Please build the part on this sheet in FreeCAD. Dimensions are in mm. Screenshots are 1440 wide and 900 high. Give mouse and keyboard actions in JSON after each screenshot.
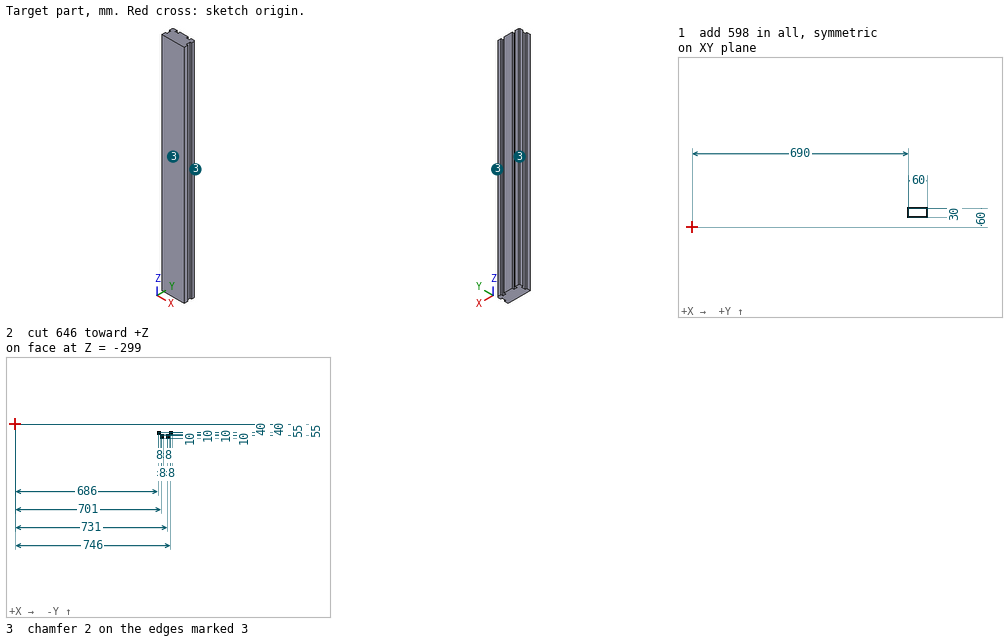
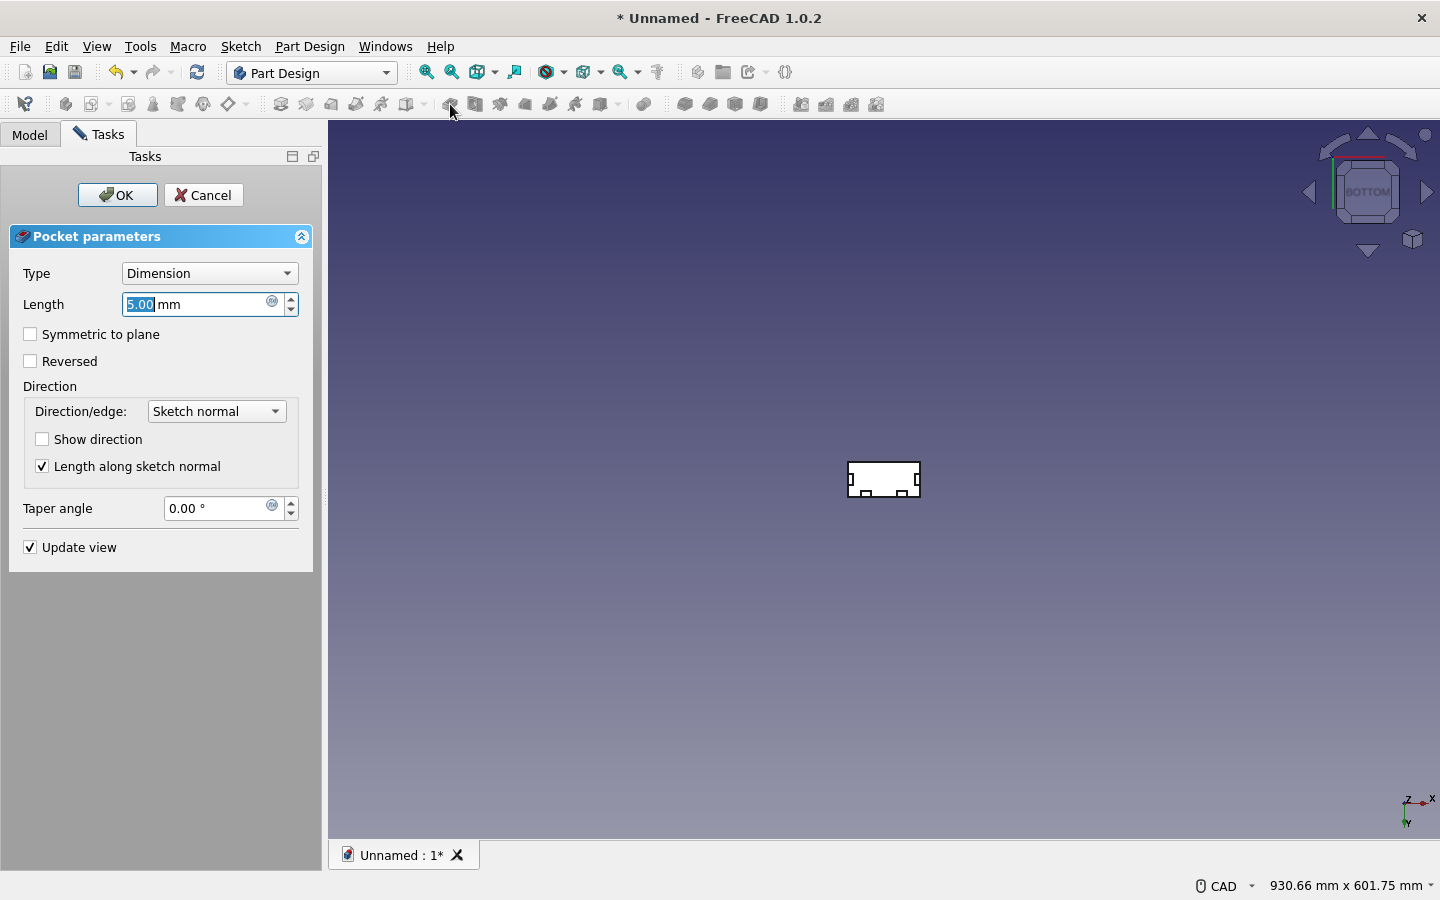
{"action": "type", "text": "646"}
{"action": "key", "text": "Tab"}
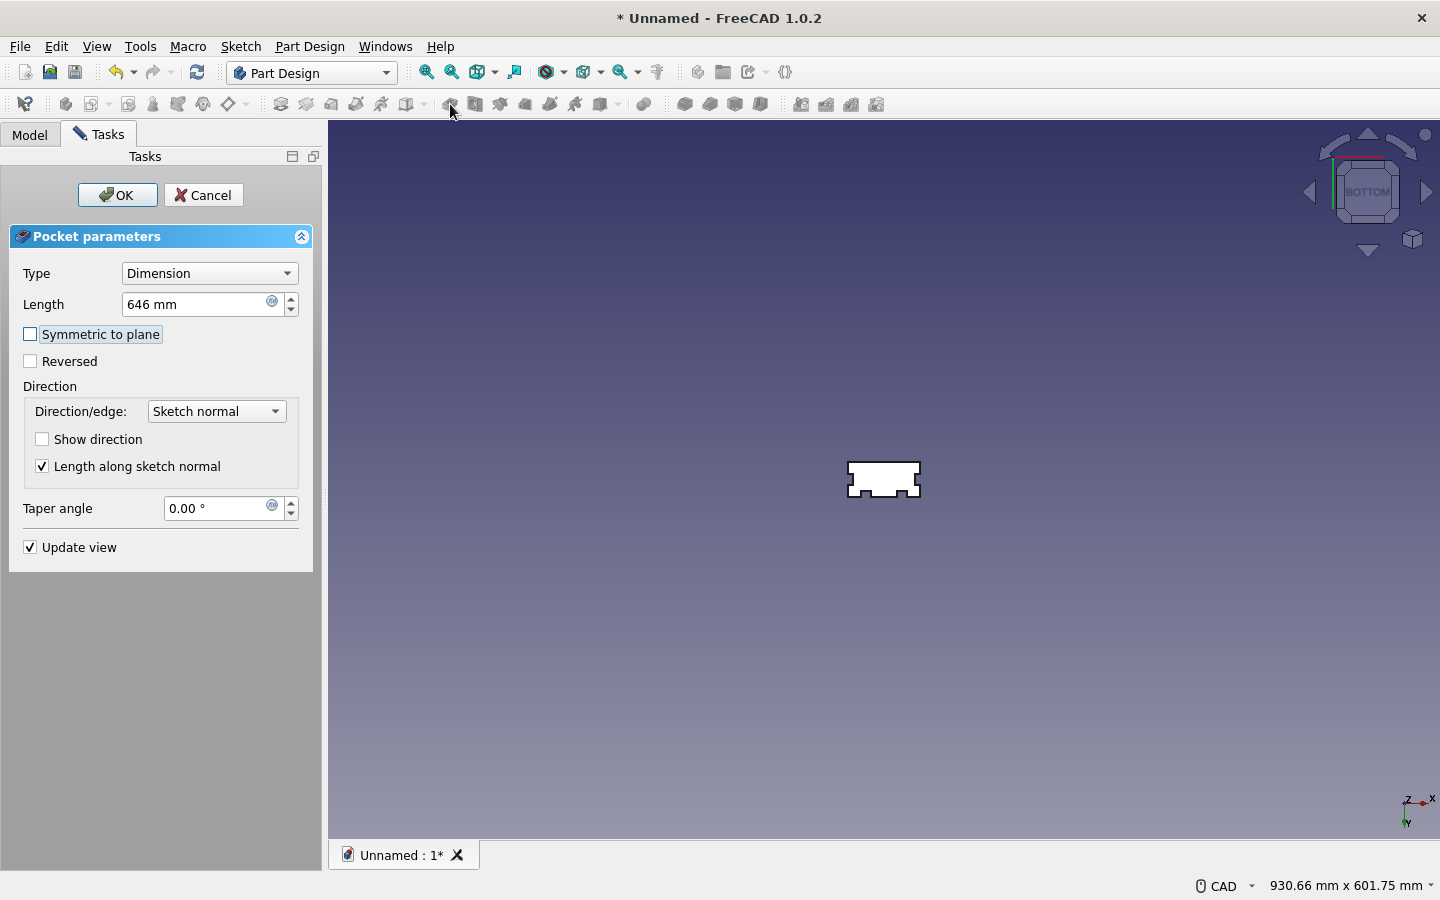
{"action": "left_click", "coordinate": [118, 195]}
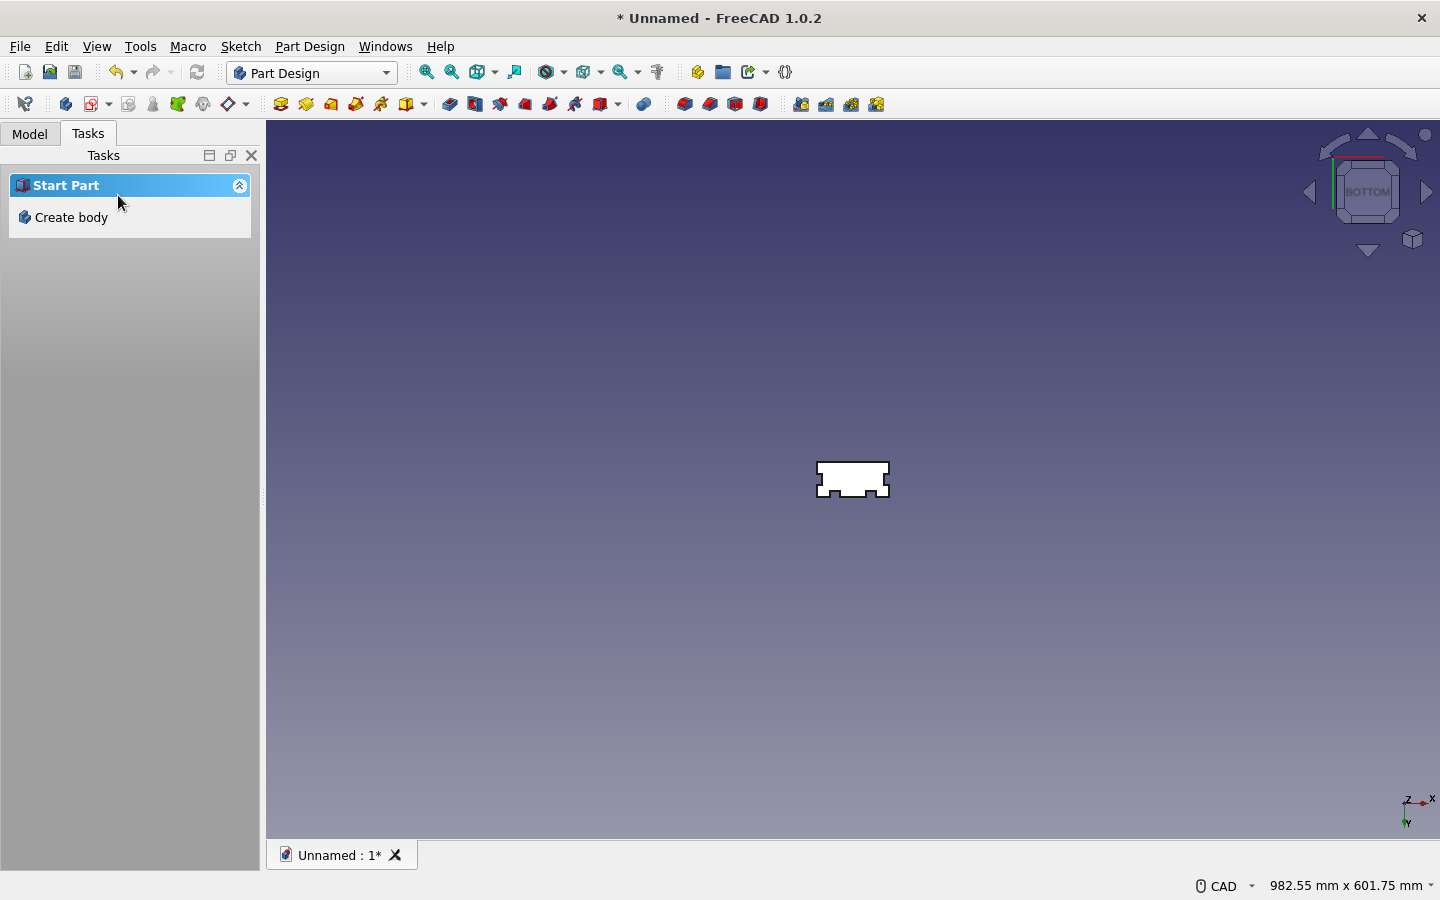
{"action": "left_click", "coordinate": [427, 72]}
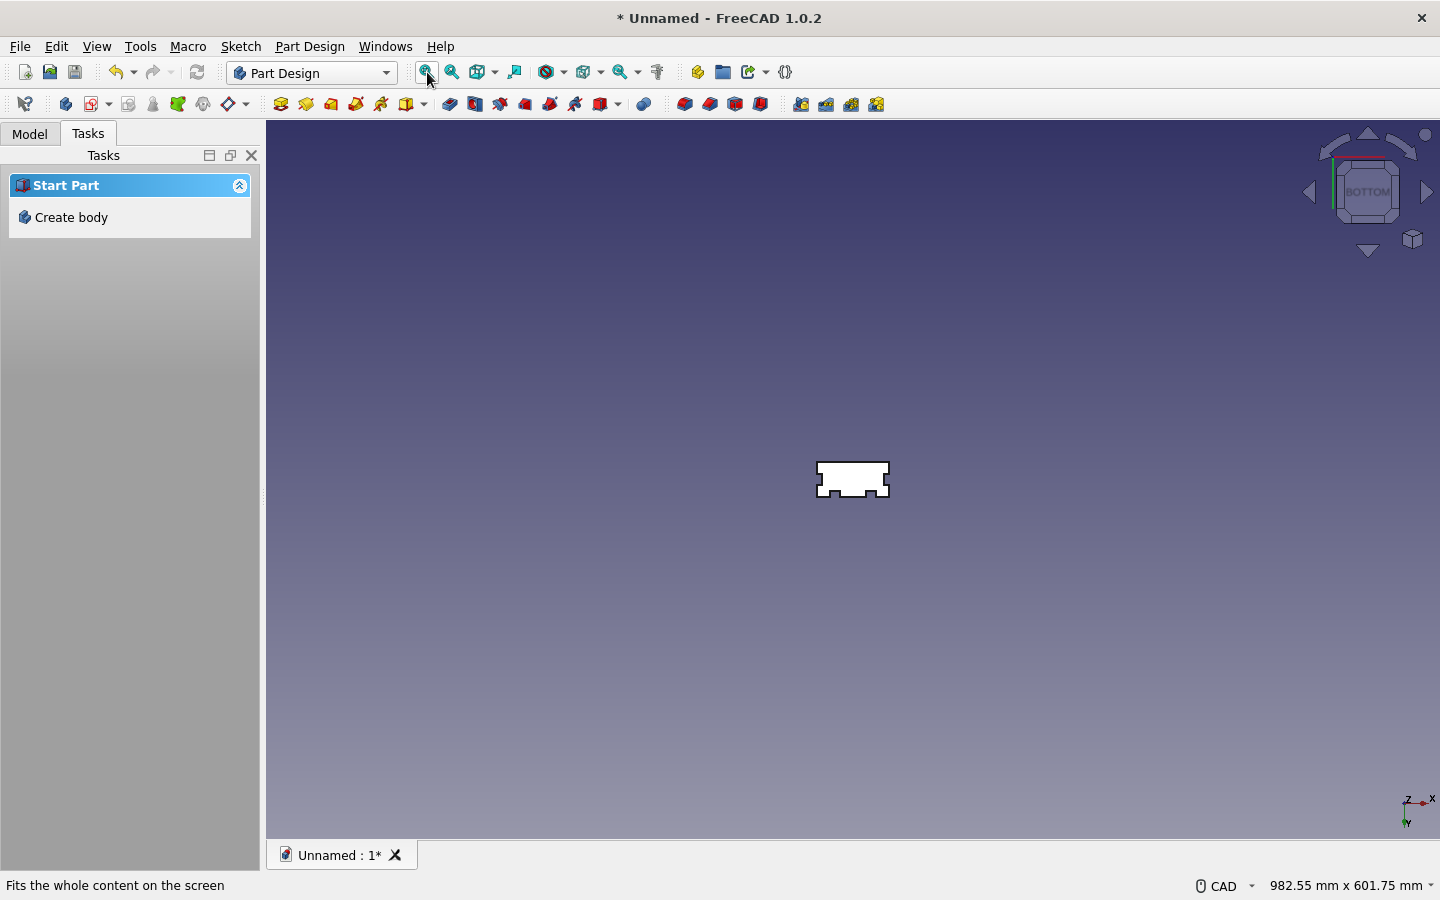
{"action": "key", "text": "0"}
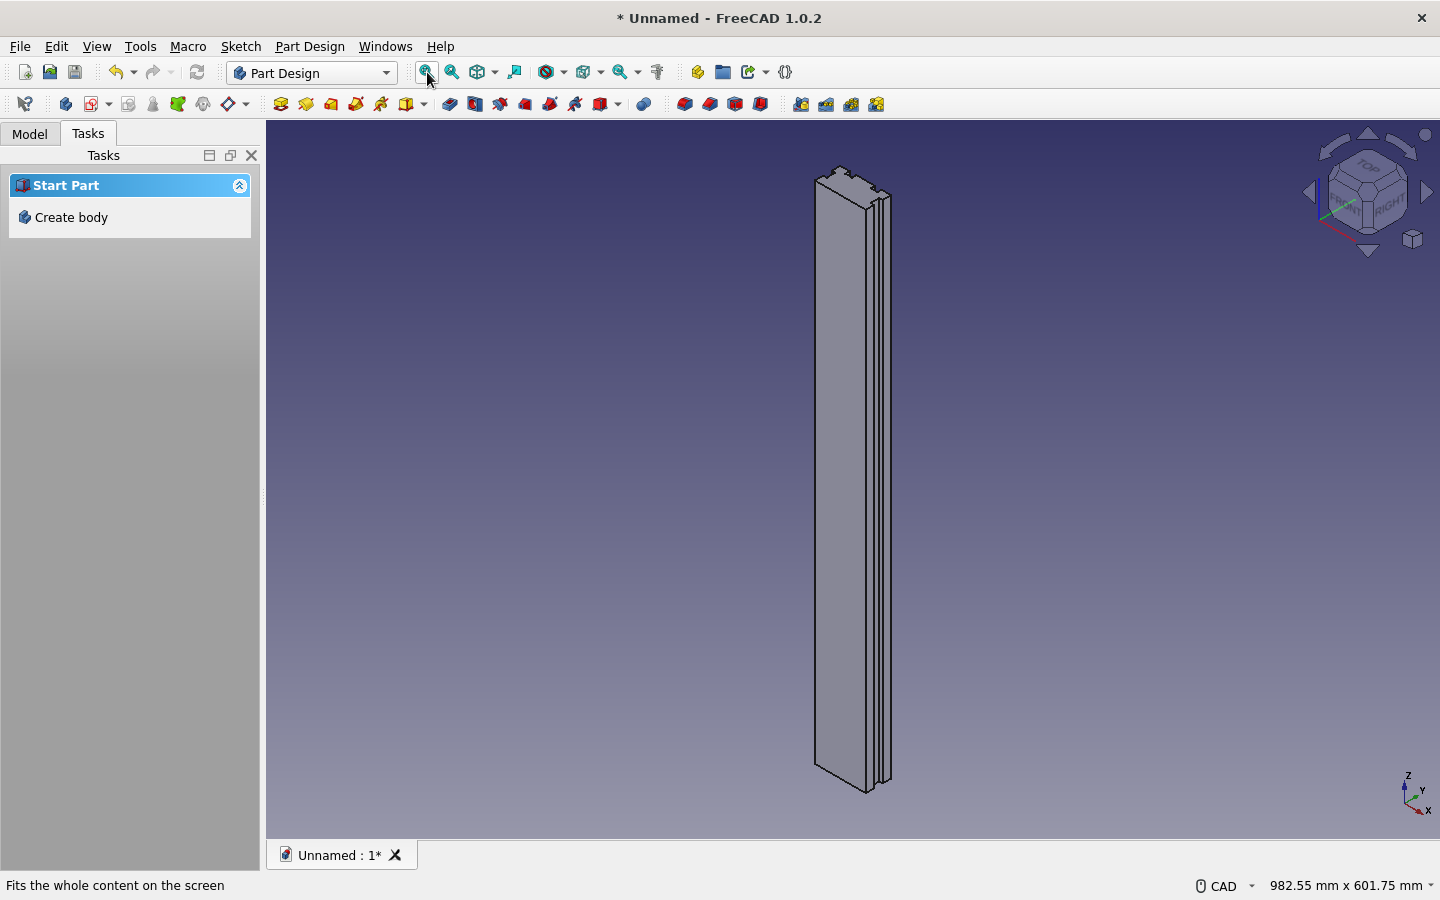
{"action": "key", "text": "2"}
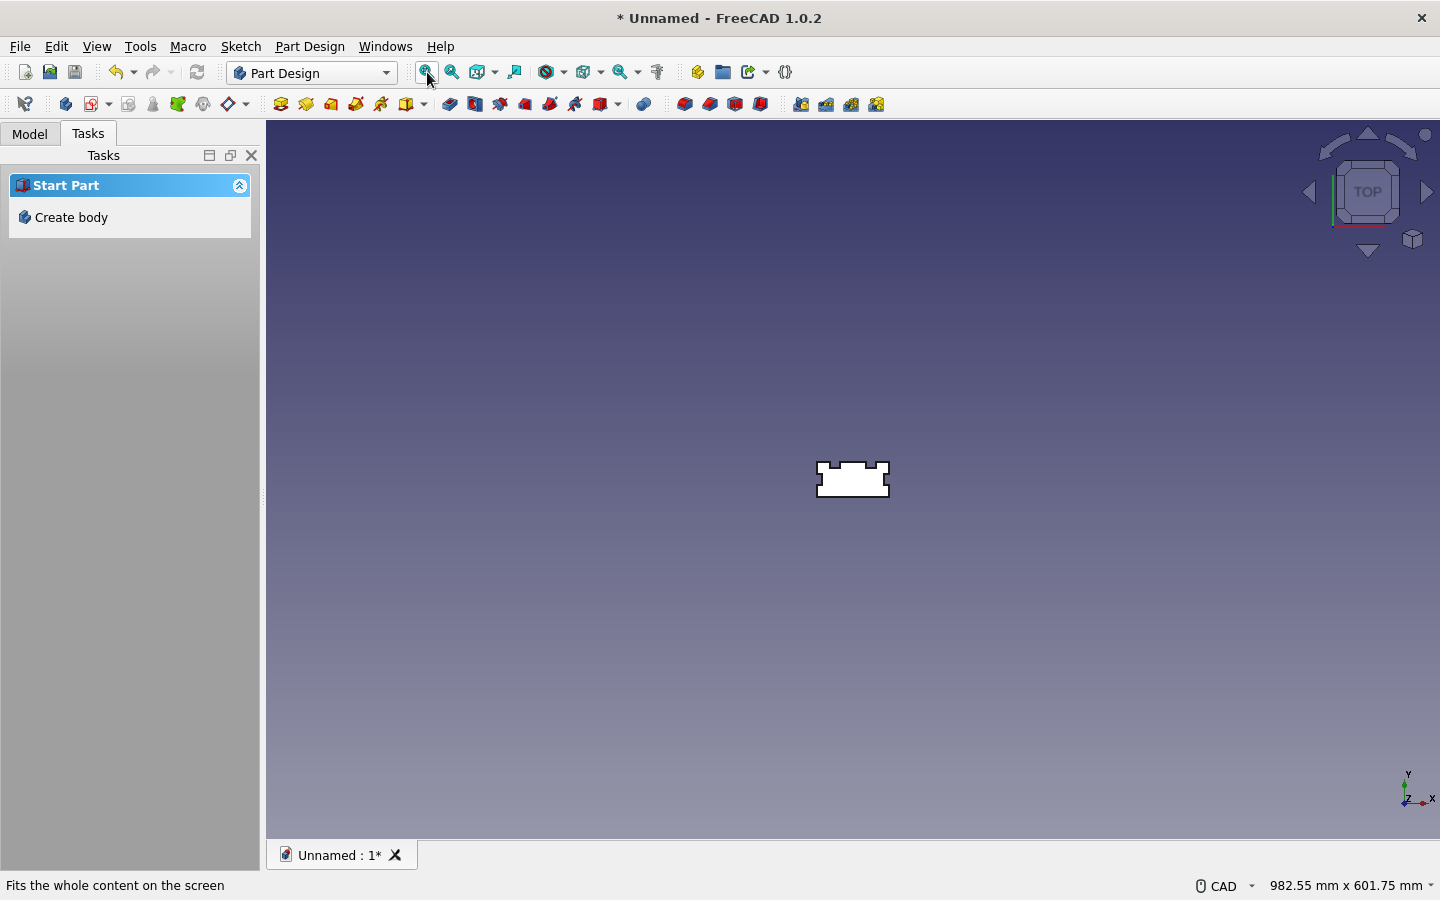
{"action": "key", "text": "v f"}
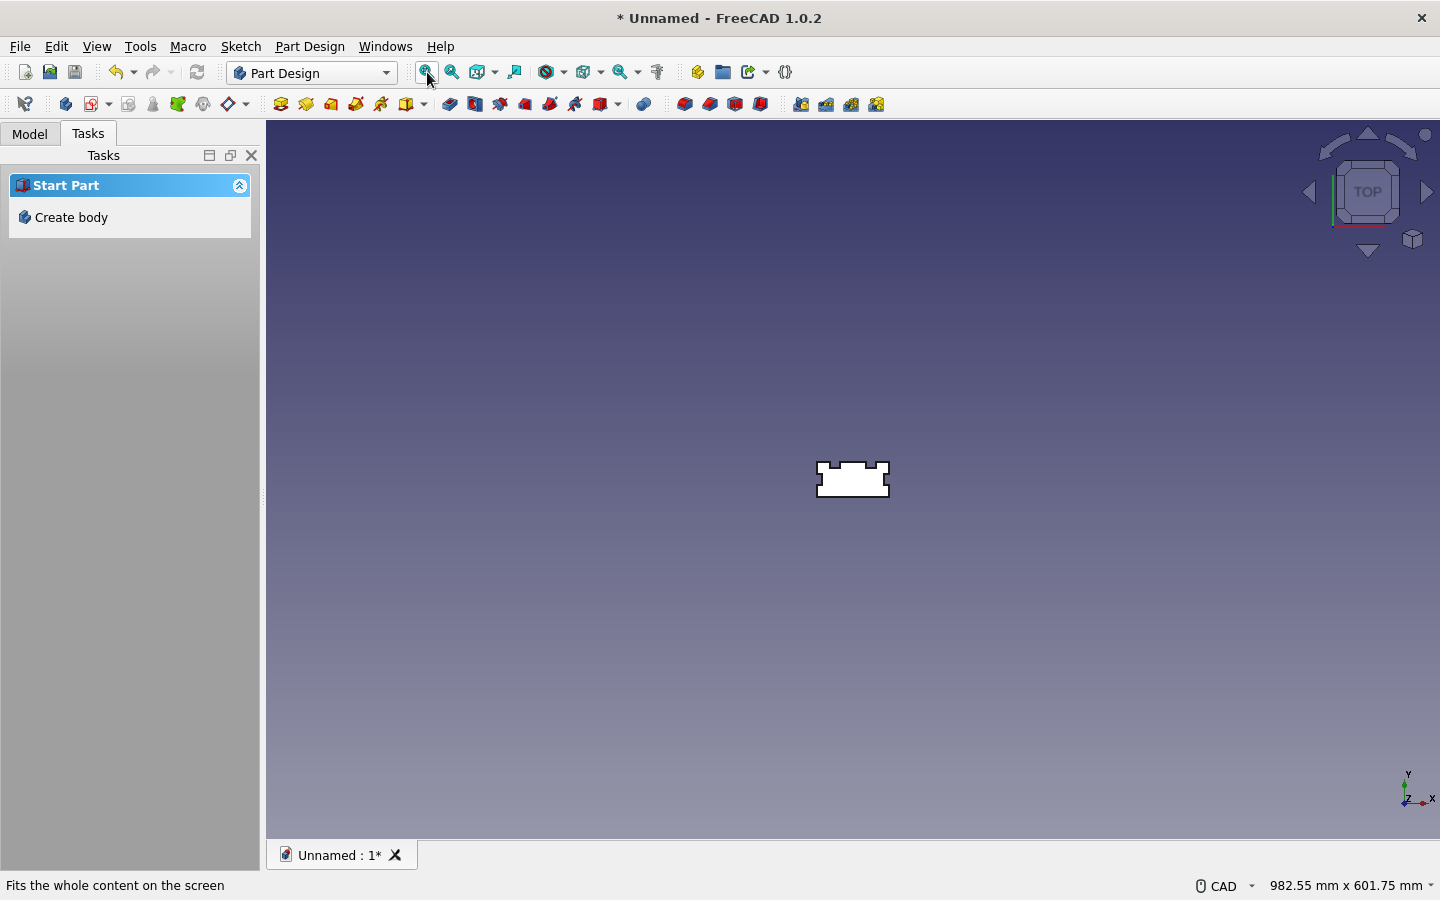
{"action": "key", "text": "1"}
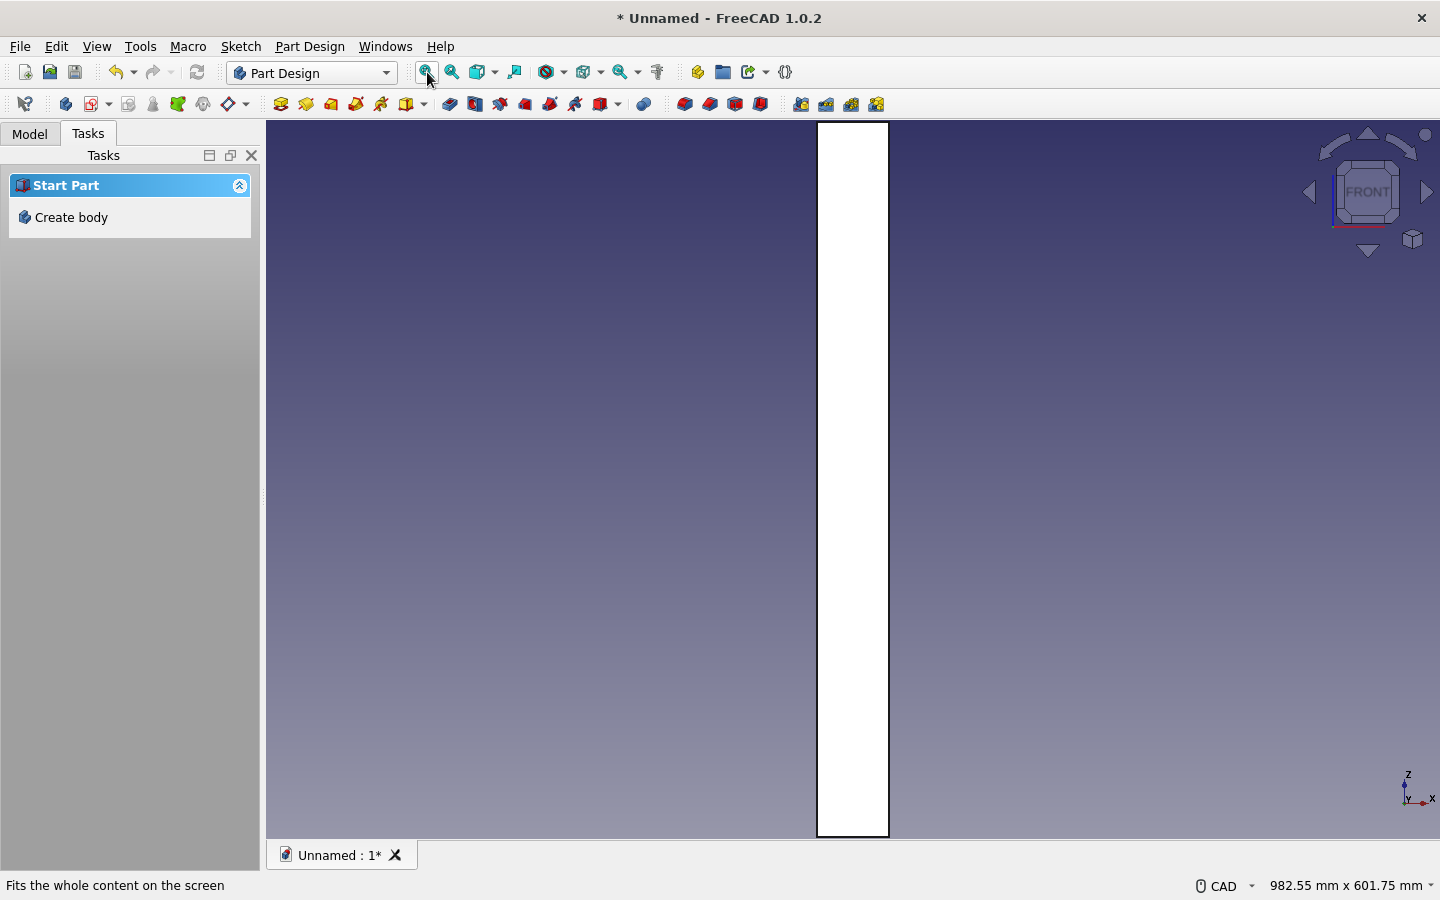
{"action": "key", "text": "3"}